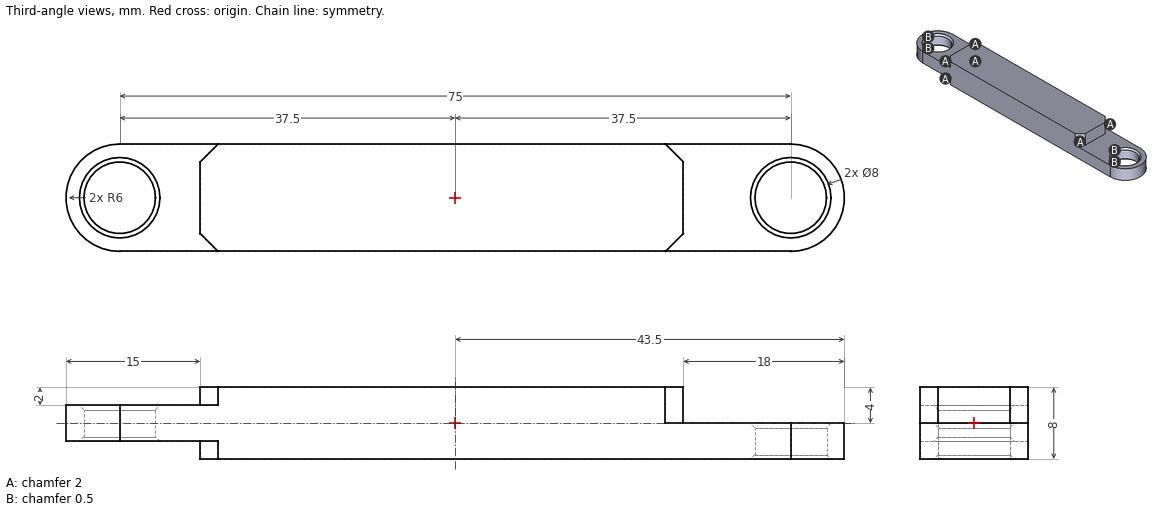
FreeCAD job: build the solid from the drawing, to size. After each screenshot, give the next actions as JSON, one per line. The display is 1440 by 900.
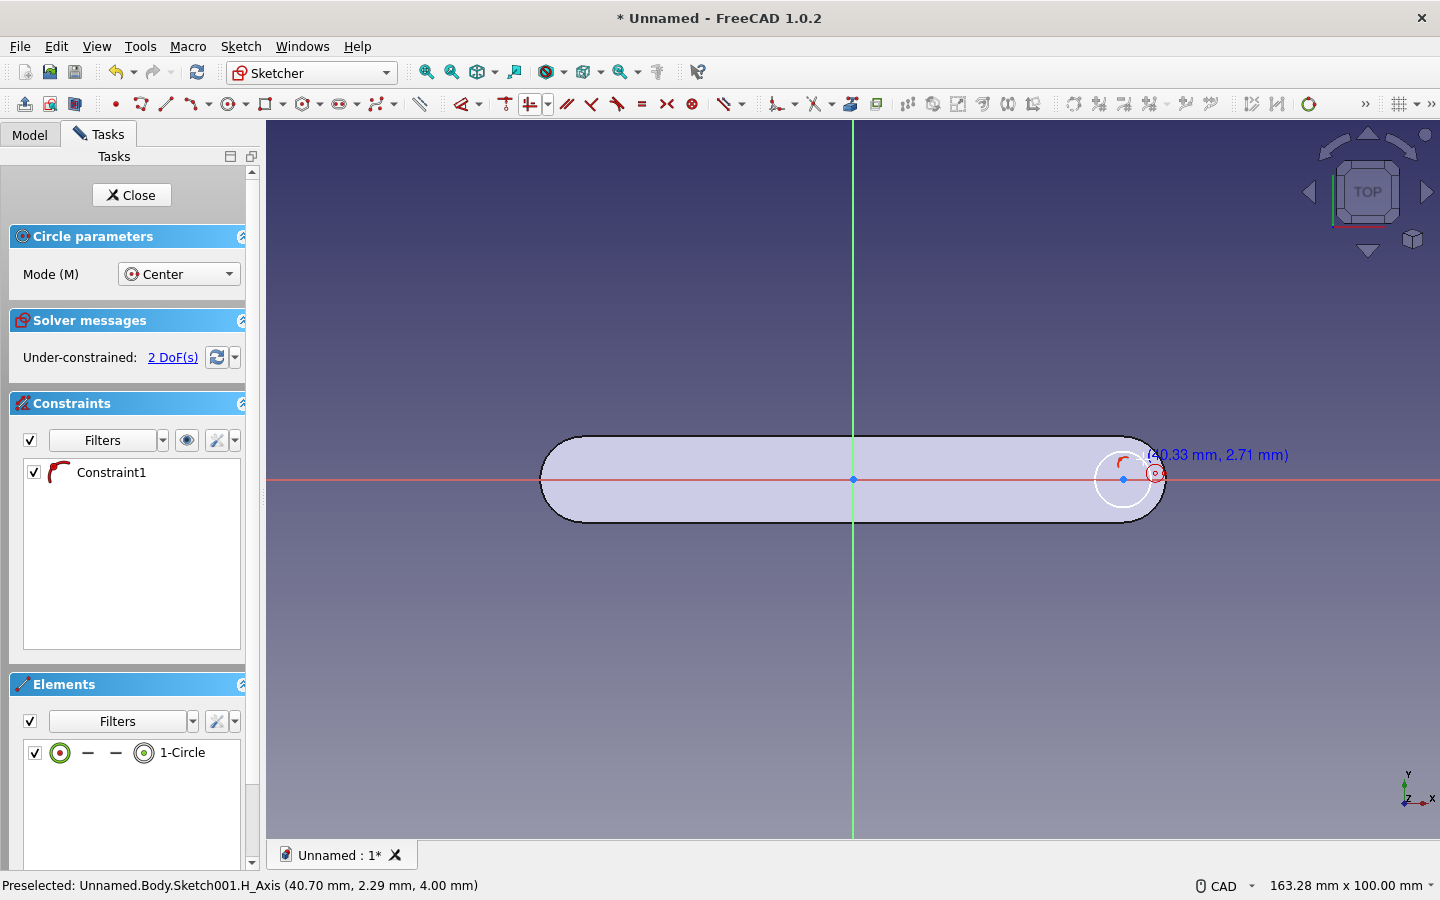
{"action": "left_click", "coordinate": [583, 480]}
{"action": "left_click", "coordinate": [604, 459]}
{"action": "key", "text": "Escape"}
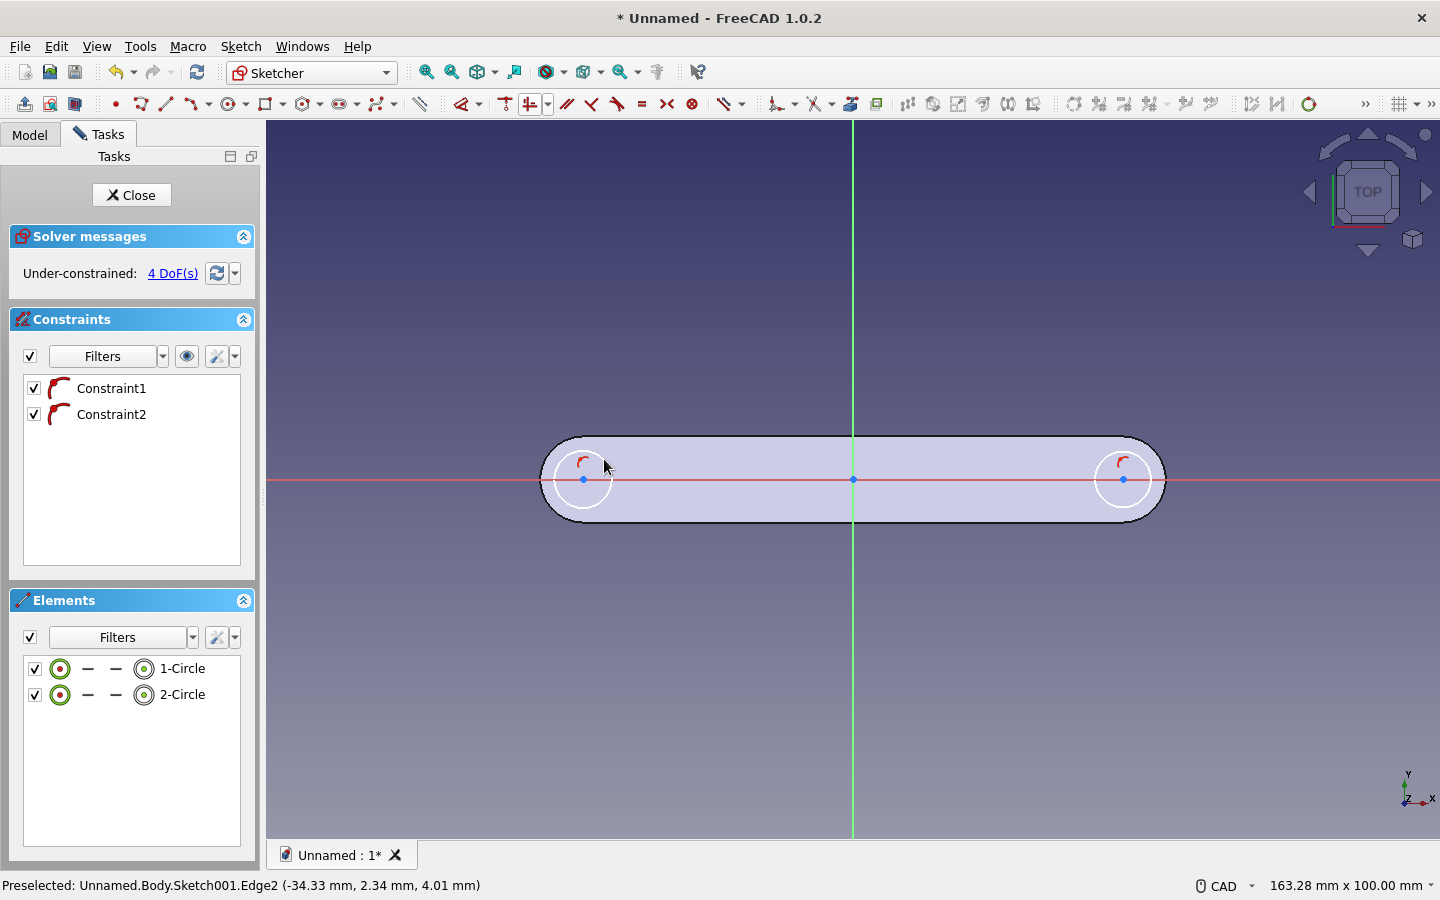
{"action": "left_click", "coordinate": [1143, 460]}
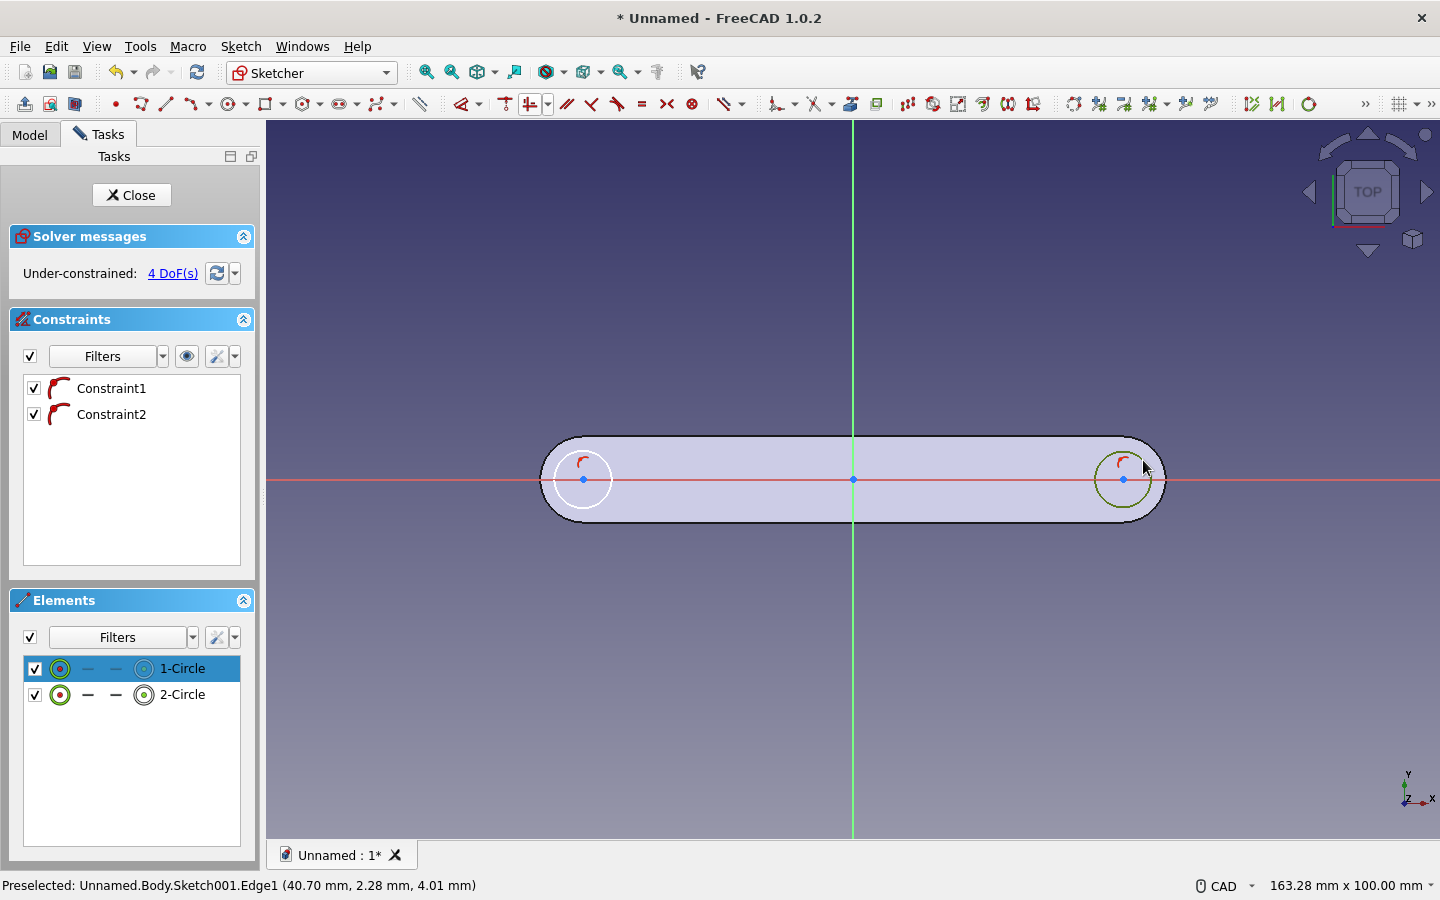
{"action": "left_click", "coordinate": [603, 459]}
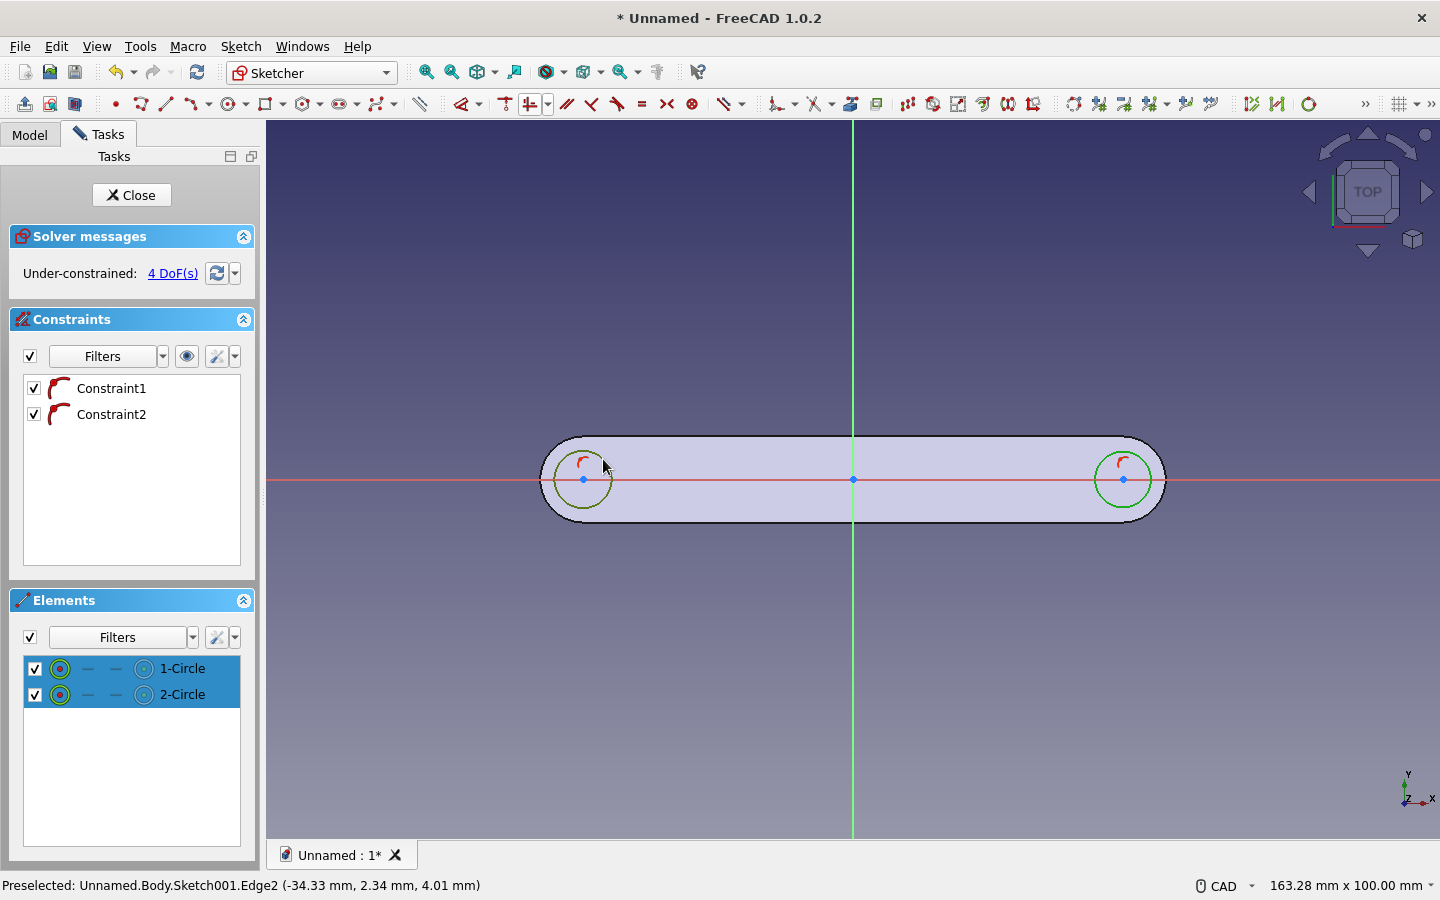
{"action": "left_click", "coordinate": [642, 104]}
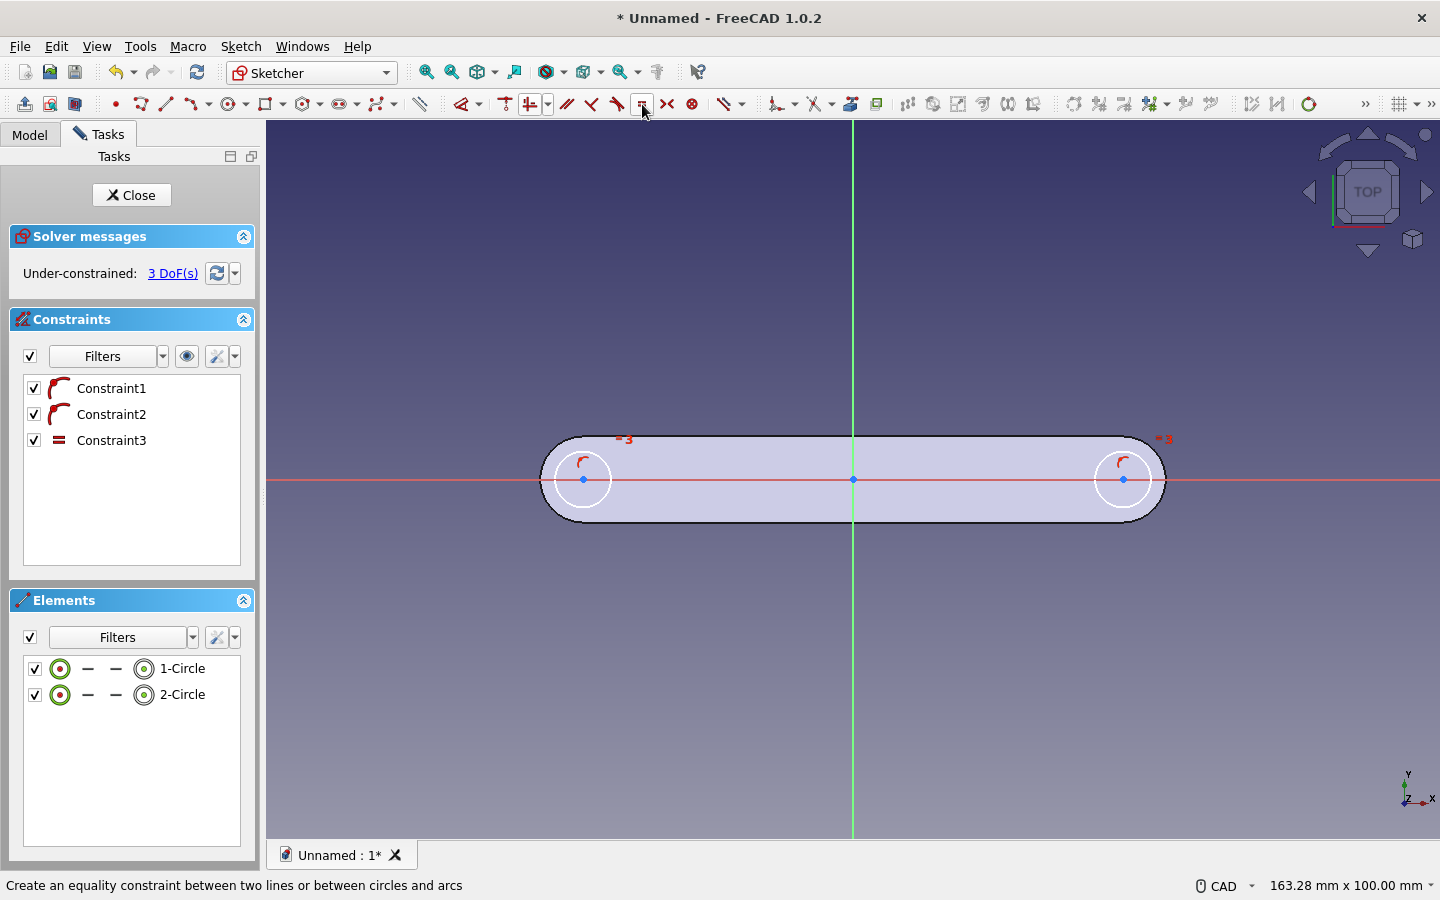
{"action": "left_click", "coordinate": [460, 104]}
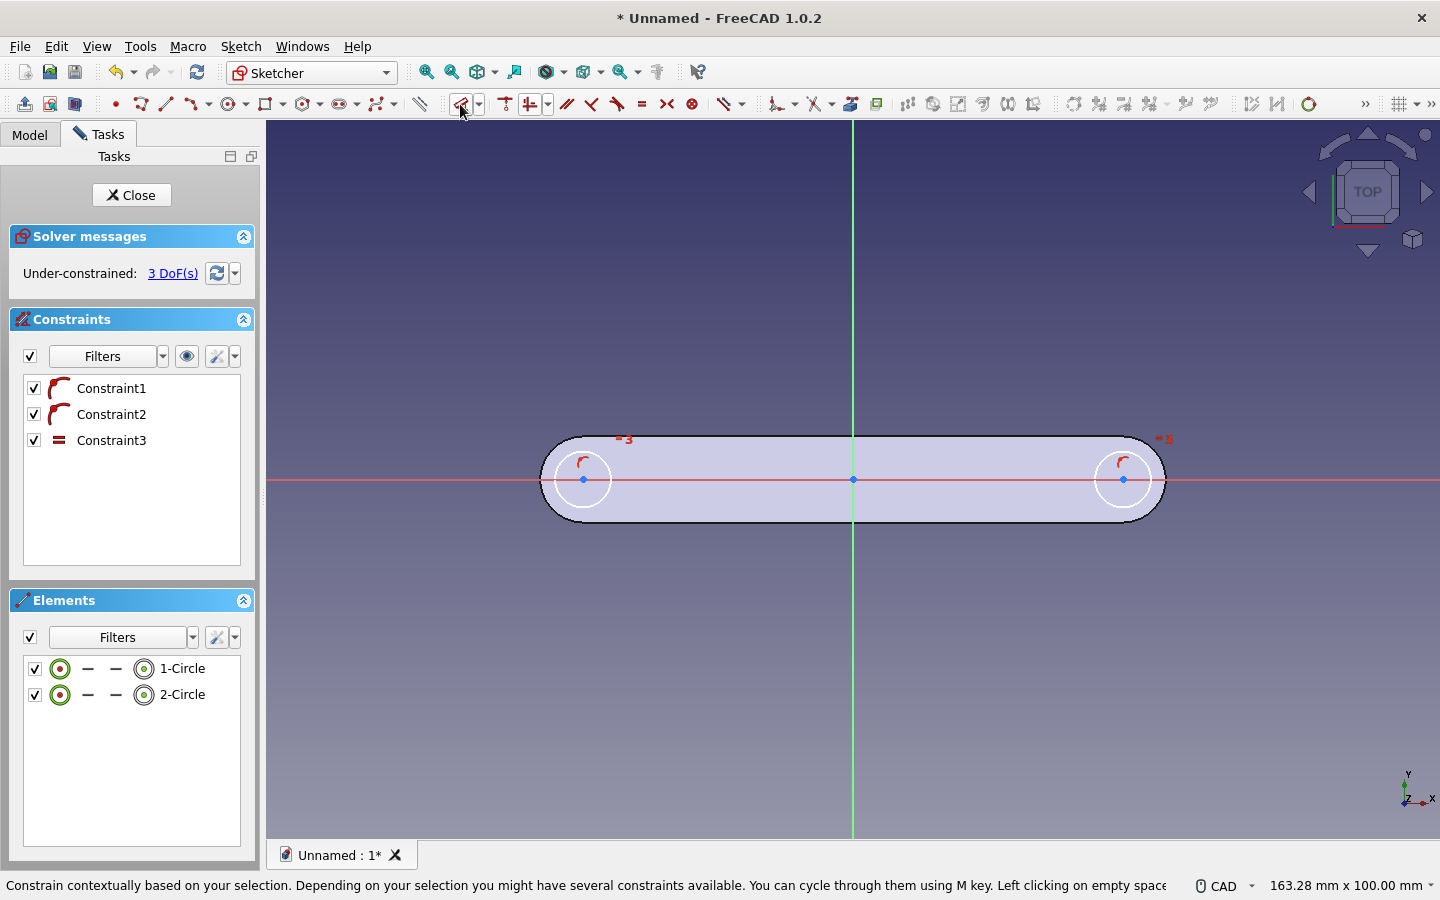
{"action": "left_click", "coordinate": [1143, 460]}
{"action": "left_click", "coordinate": [1166, 438]}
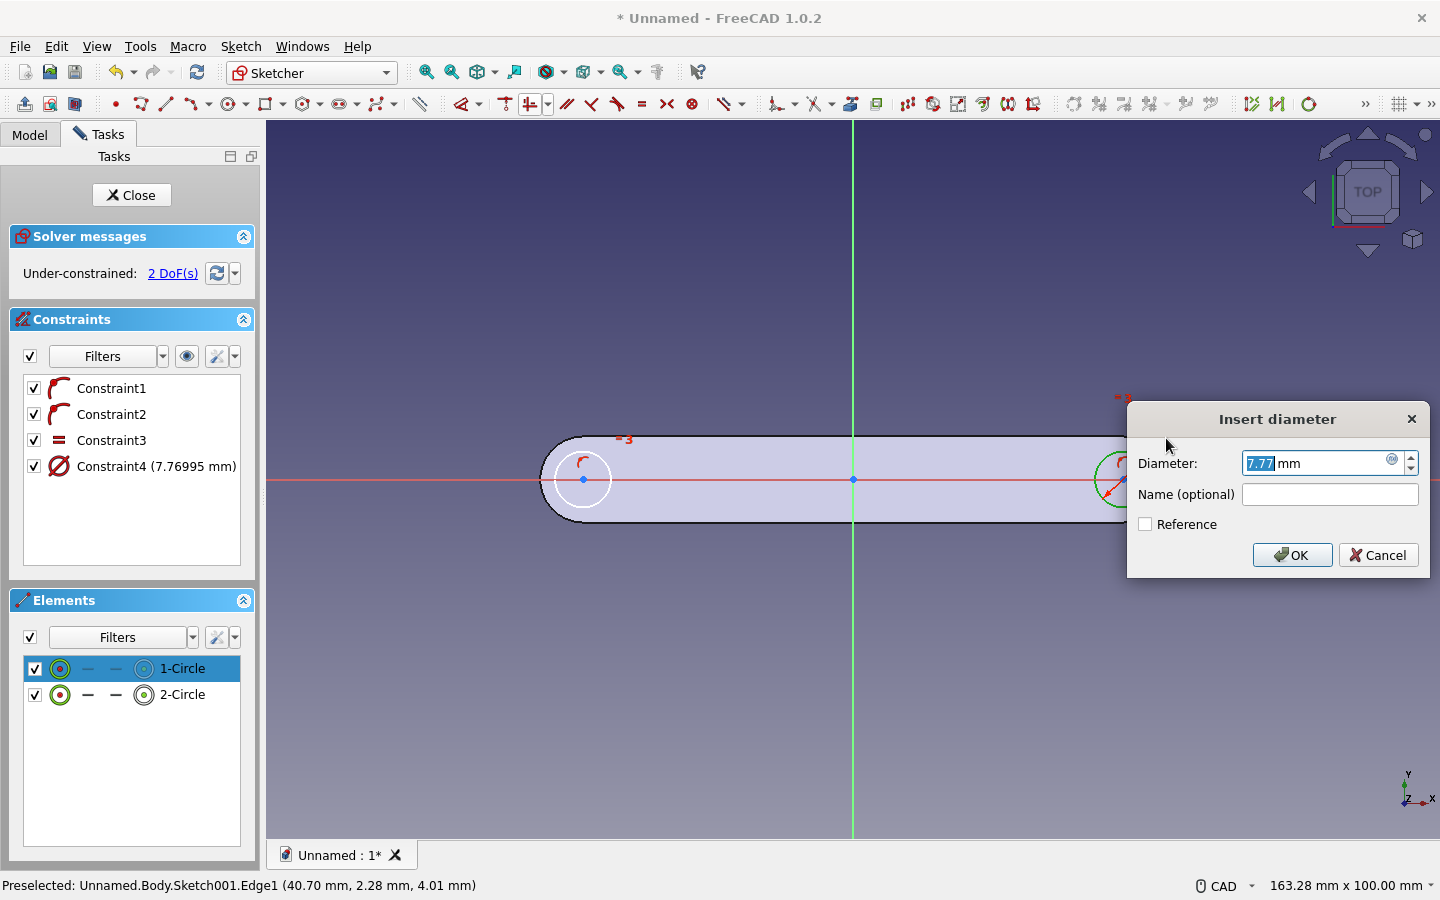
{"action": "type", "text": "8"}
{"action": "key", "text": "Return"}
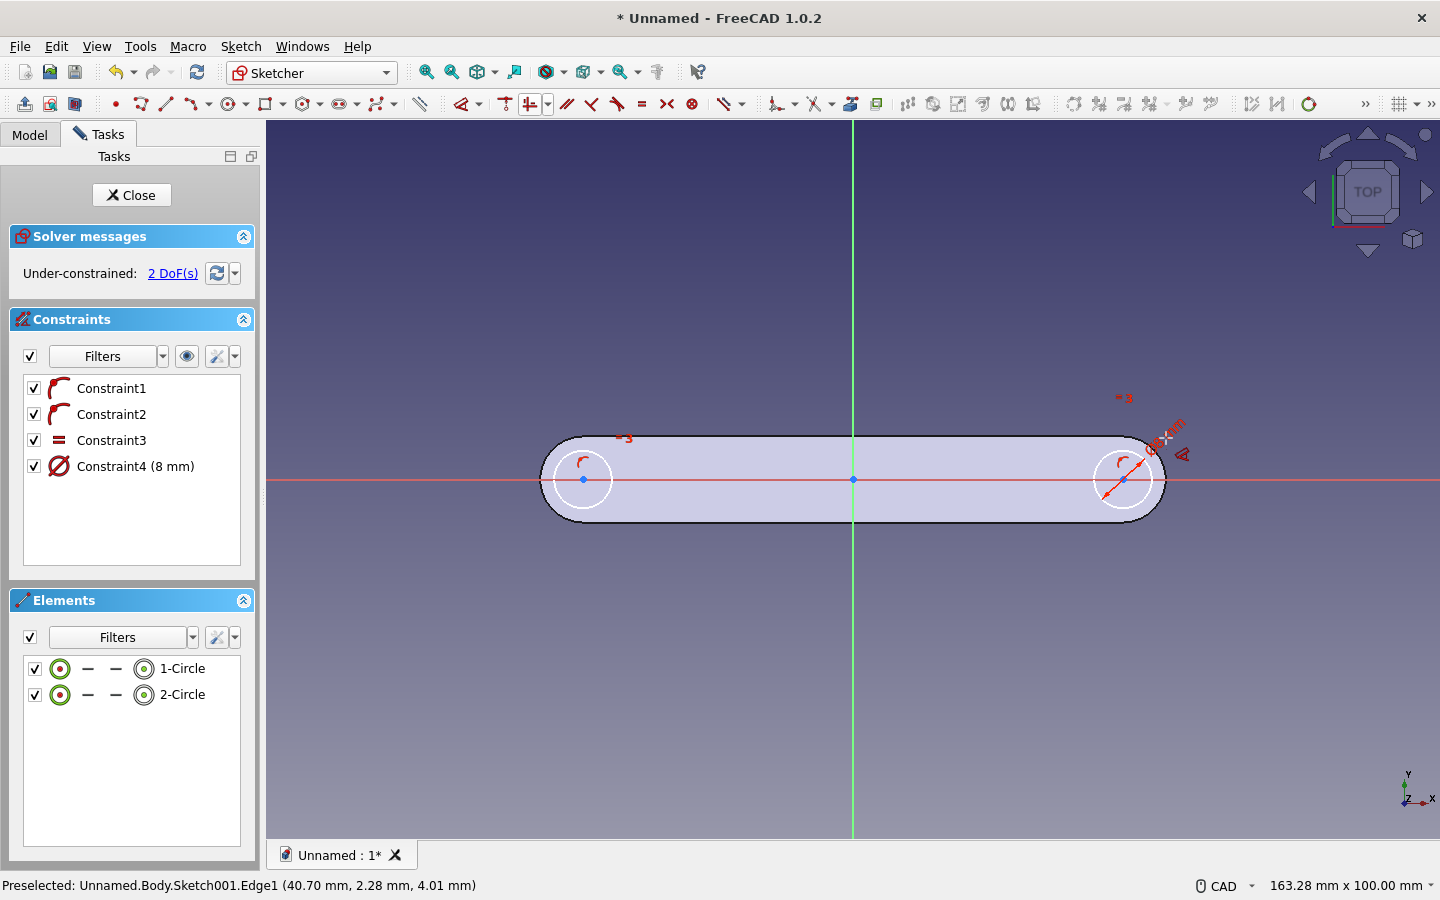
{"action": "left_click", "coordinate": [1123, 480]}